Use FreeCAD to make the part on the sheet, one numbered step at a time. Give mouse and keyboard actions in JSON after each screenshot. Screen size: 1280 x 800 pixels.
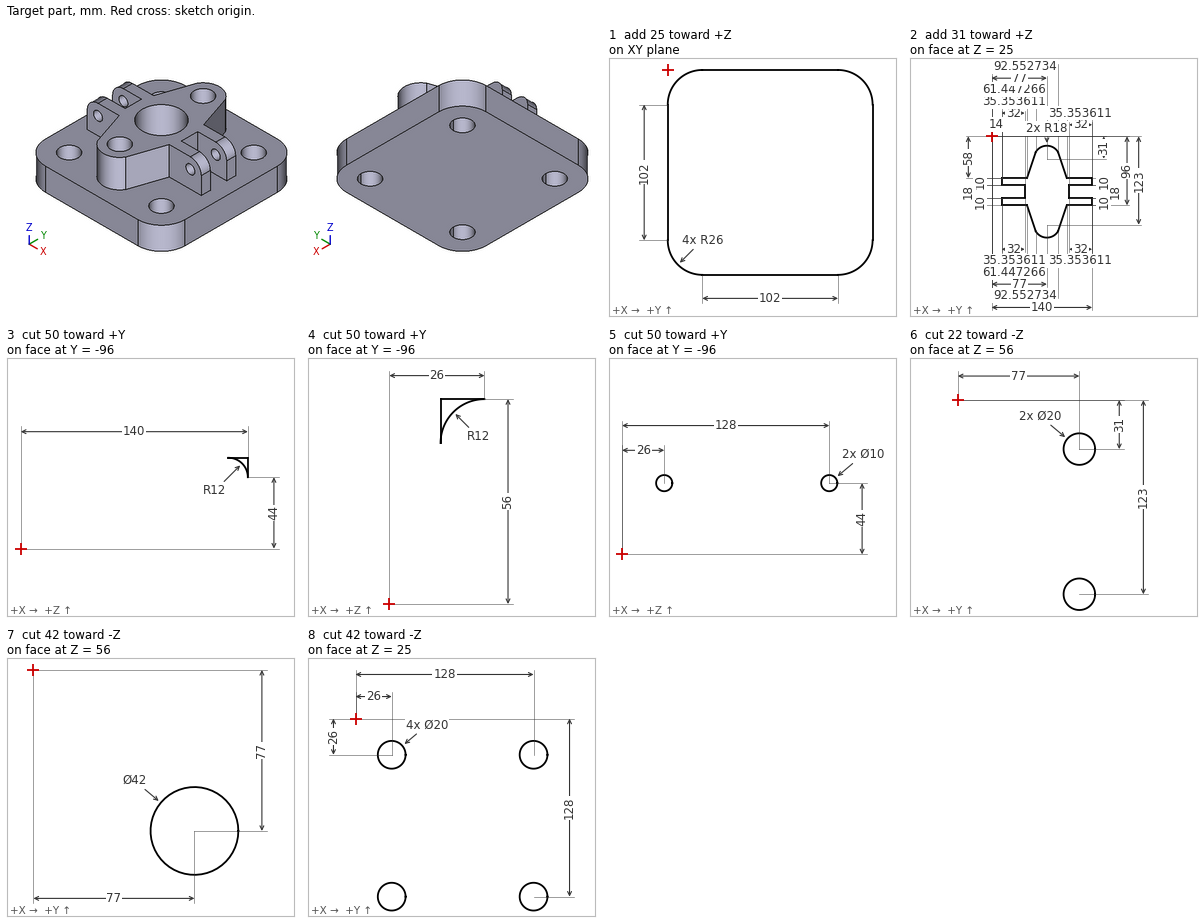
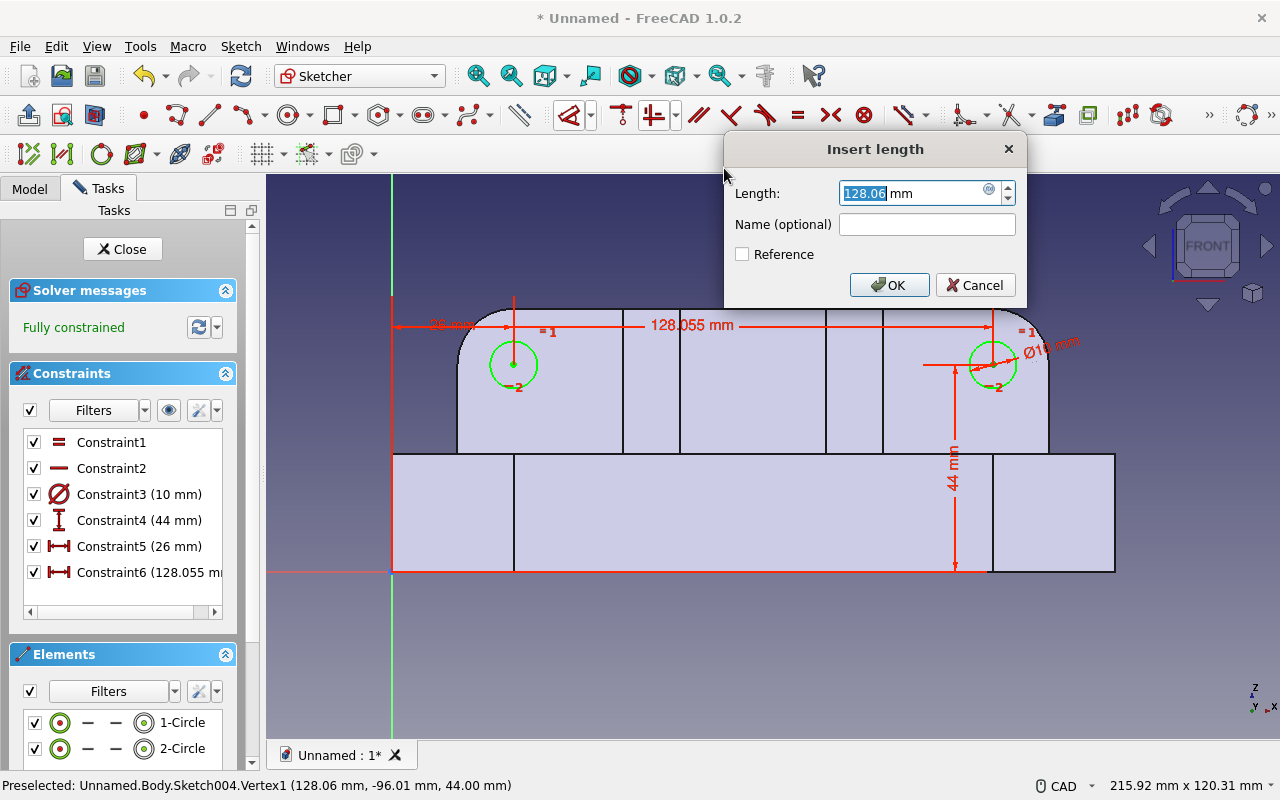
{"action": "type", "text": "128"}
{"action": "key", "text": "Return"}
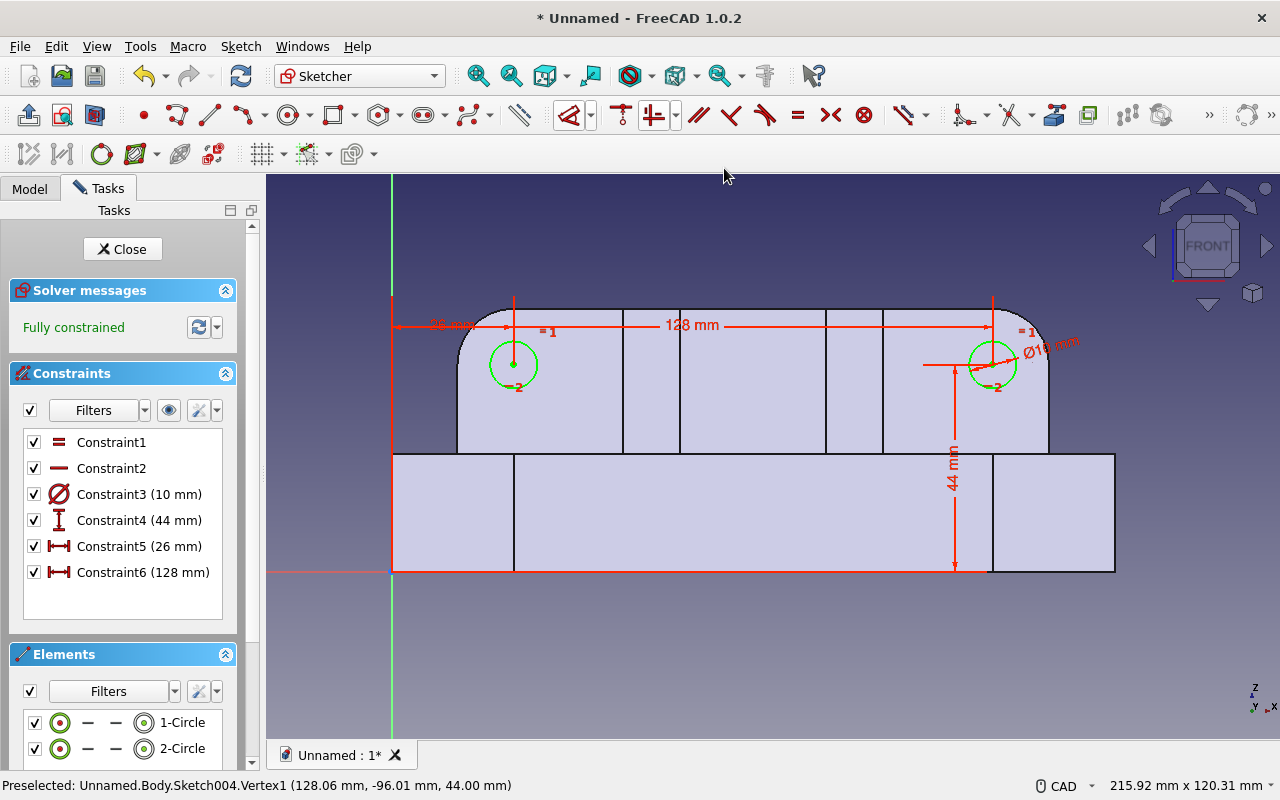
{"action": "left_click", "coordinate": [123, 249]}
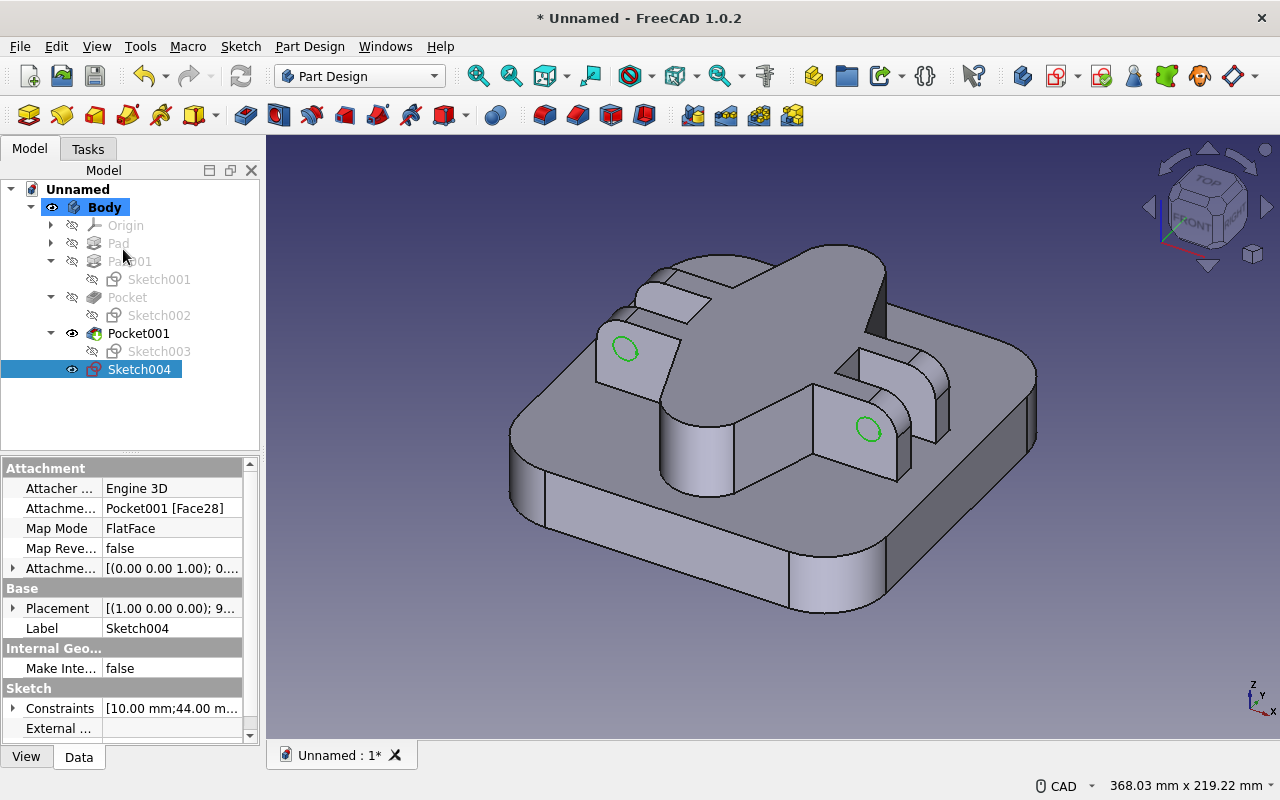
{"action": "left_click", "coordinate": [246, 116]}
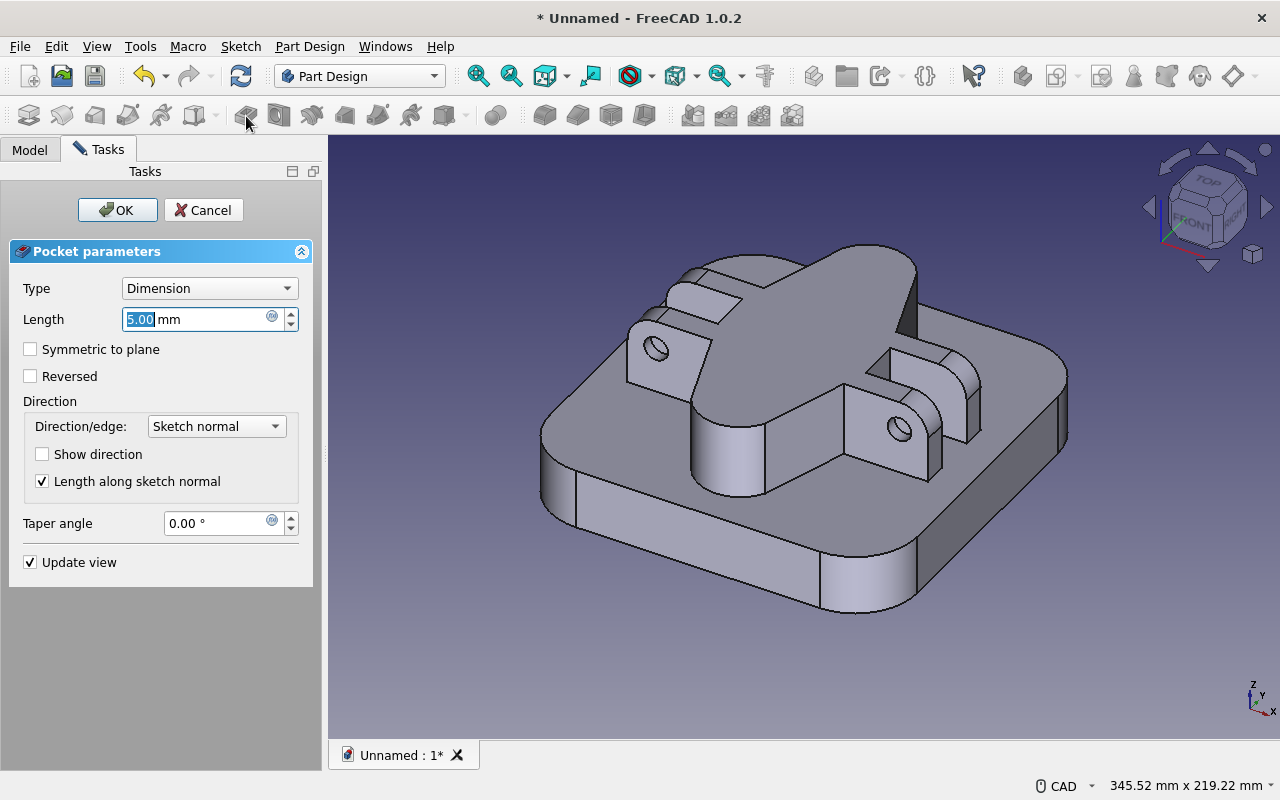
{"action": "type", "text": "50"}
{"action": "key", "text": "Tab"}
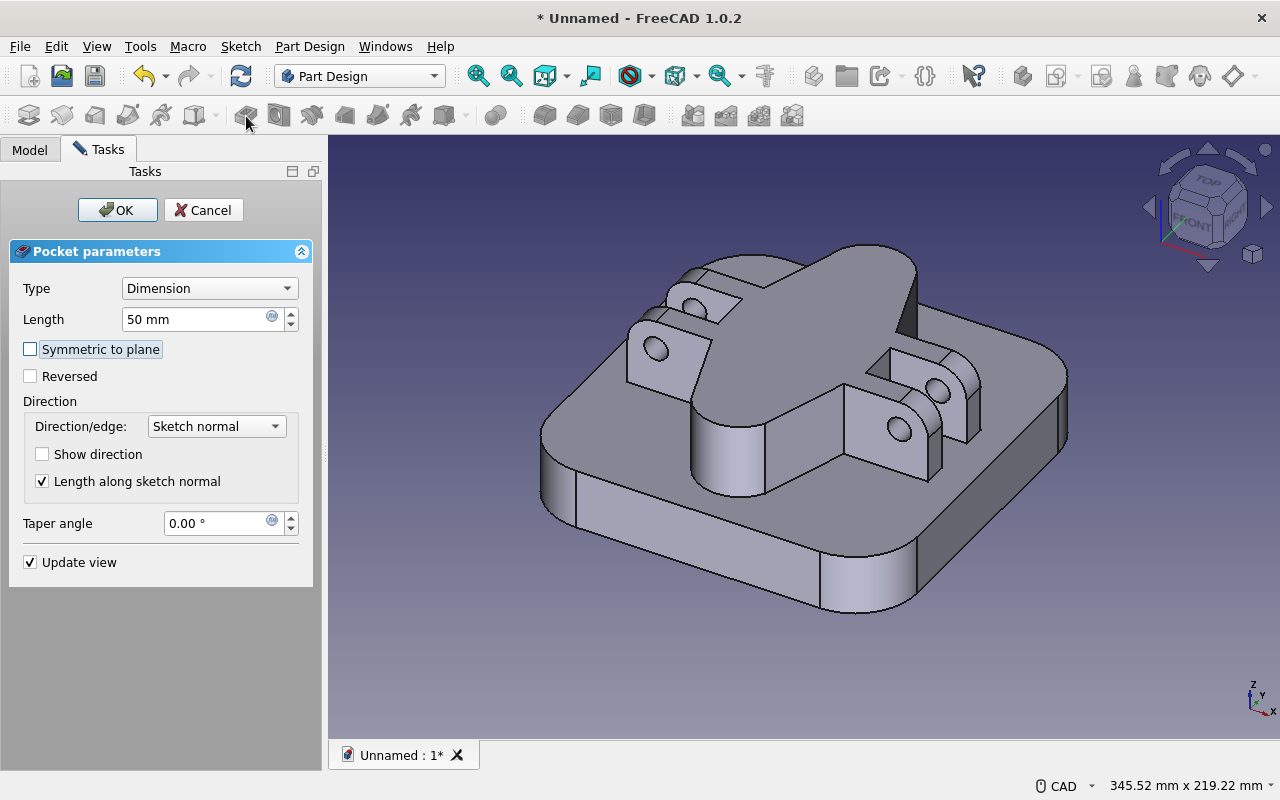
{"action": "left_click", "coordinate": [118, 210]}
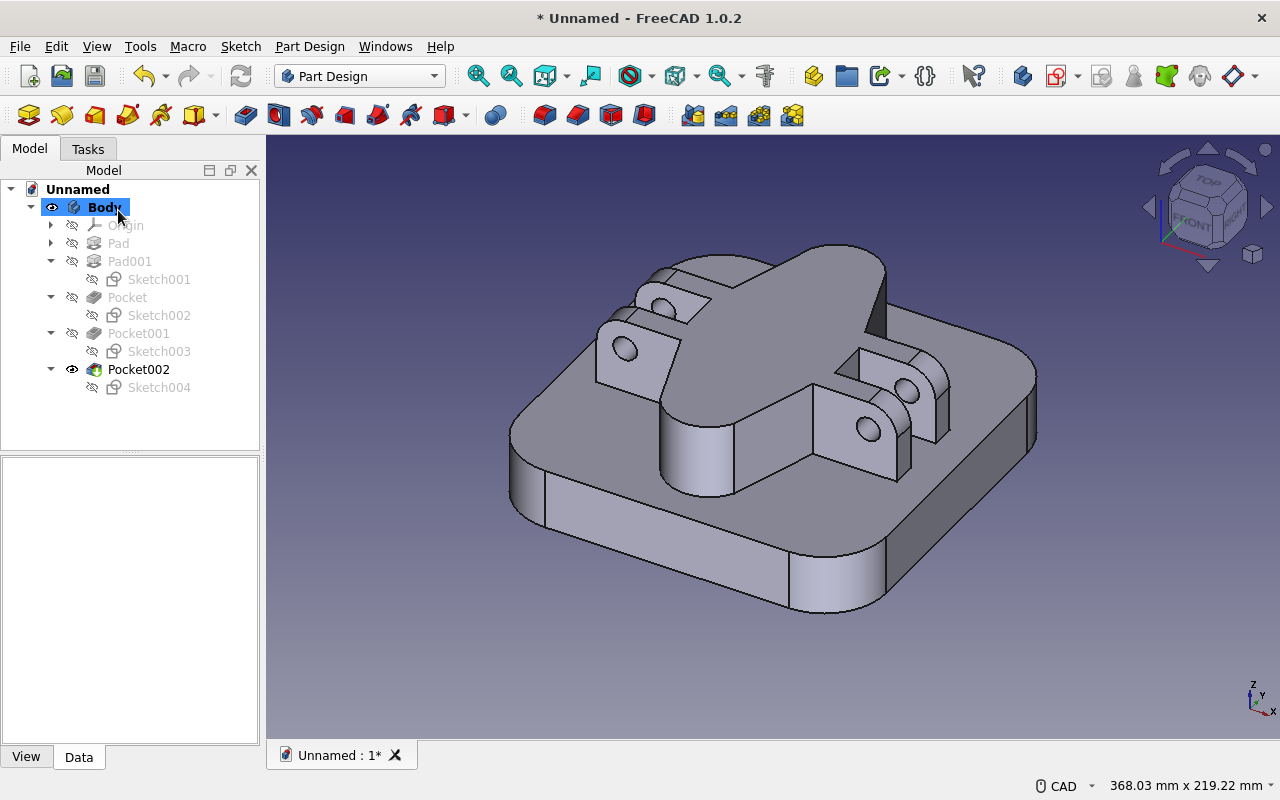
{"action": "left_click", "coordinate": [773, 335]}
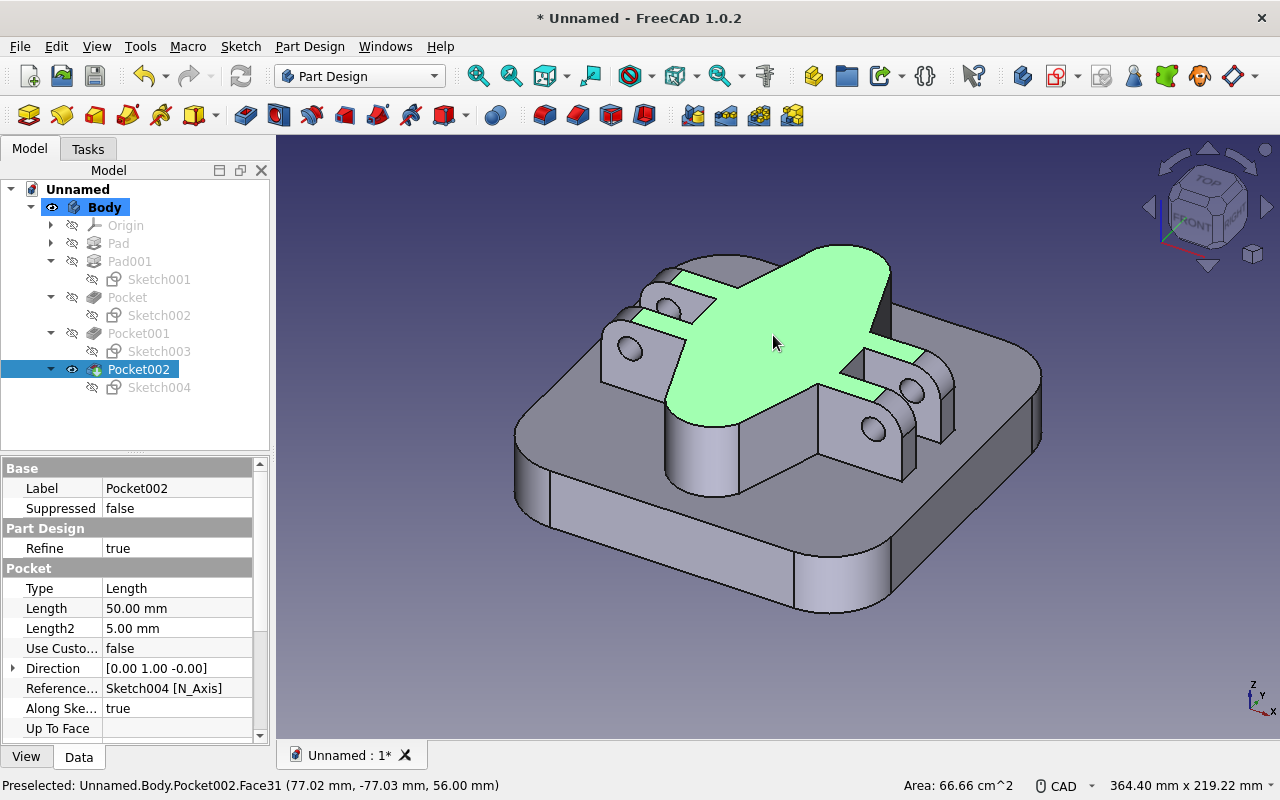
{"action": "left_click", "coordinate": [1056, 76]}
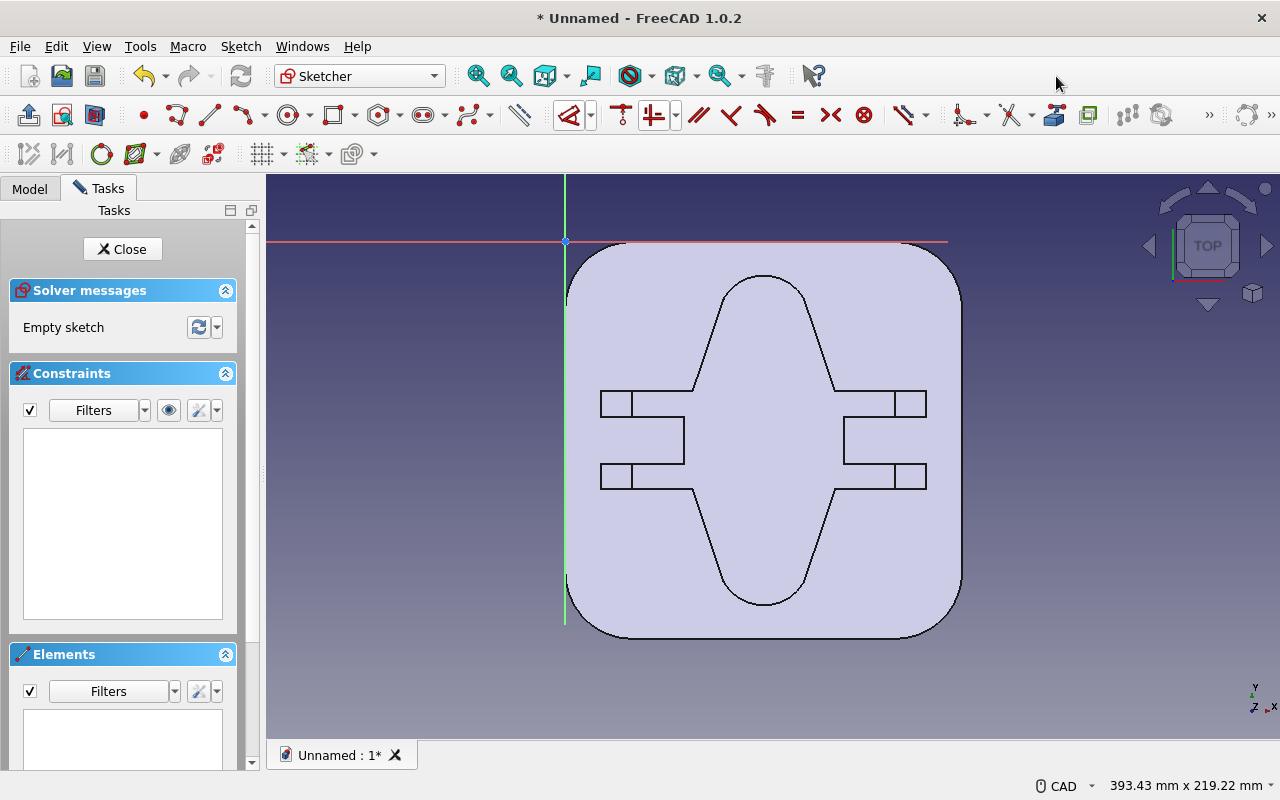
{"action": "left_click", "coordinate": [288, 116]}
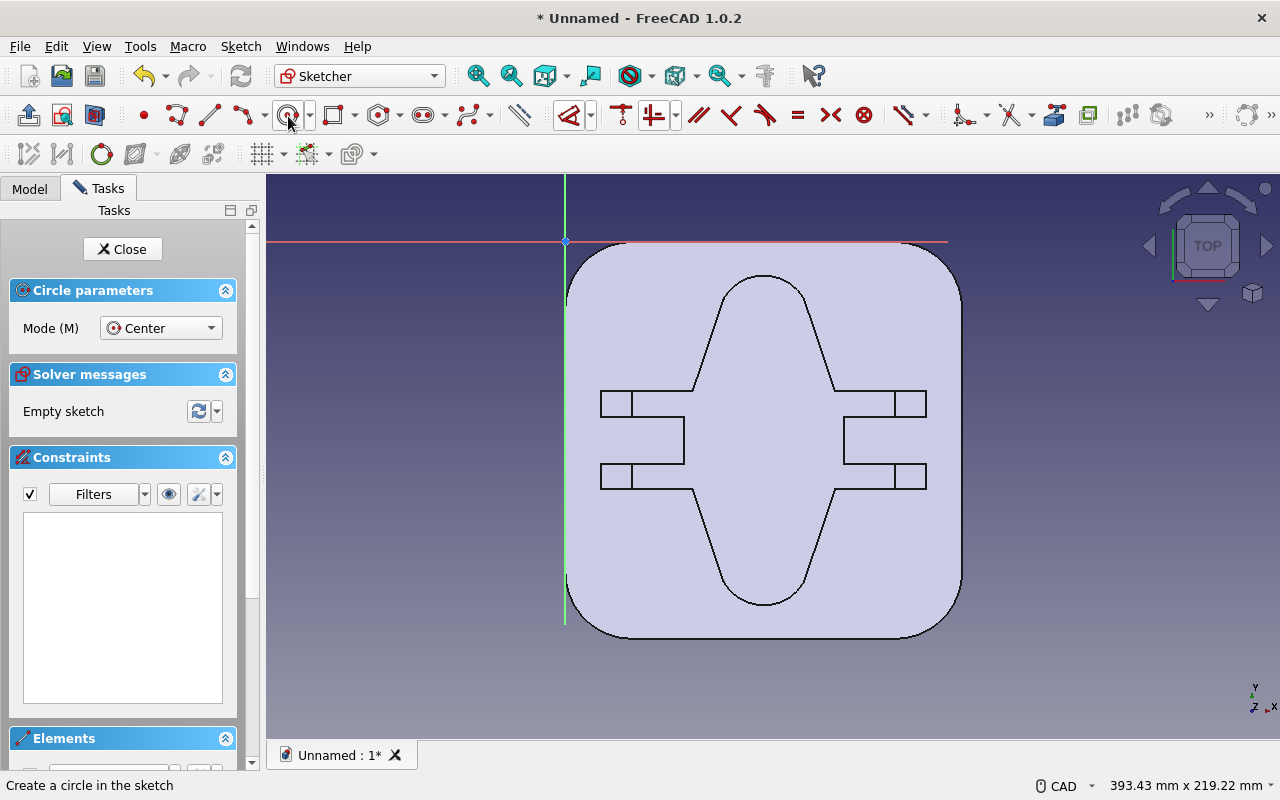
{"action": "left_click", "coordinate": [764, 322]}
{"action": "left_click", "coordinate": [782, 304]}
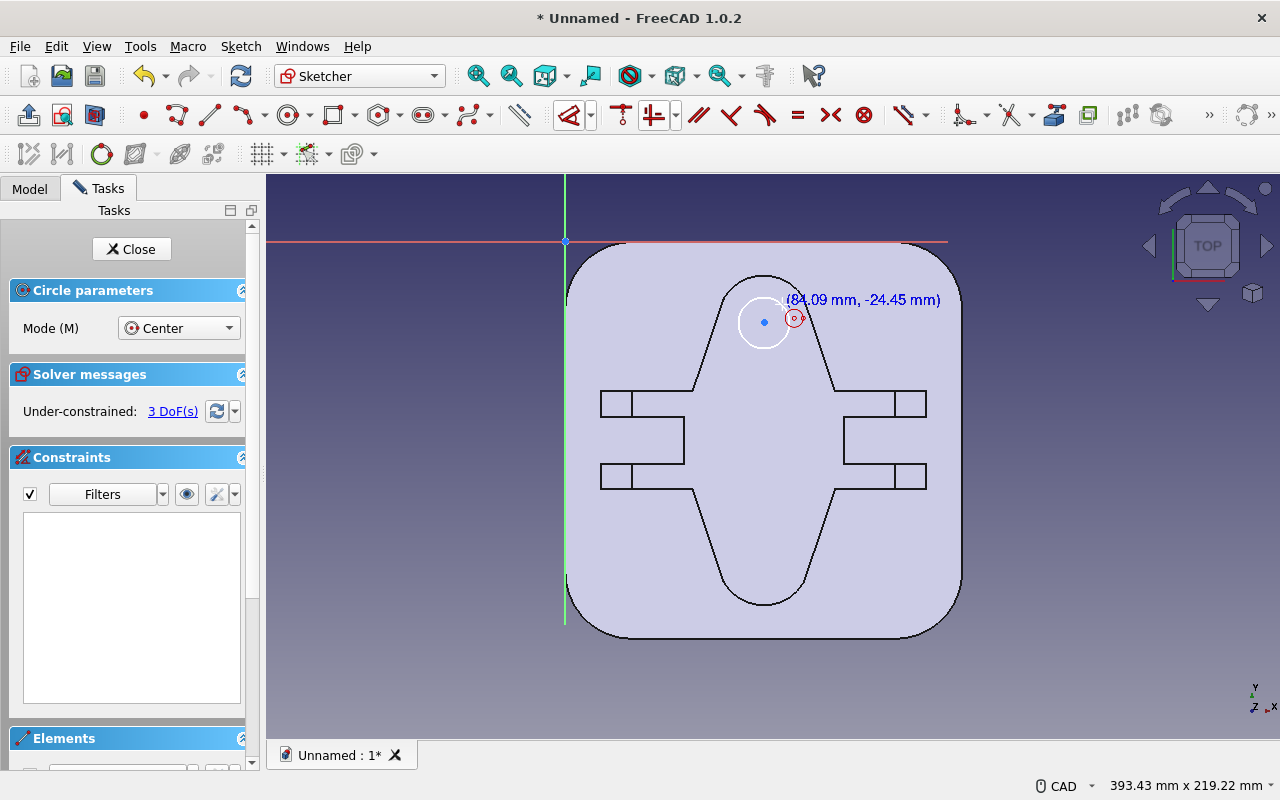
{"action": "left_click", "coordinate": [764, 559]}
{"action": "left_click", "coordinate": [782, 541]}
{"action": "key", "text": "Escape"}